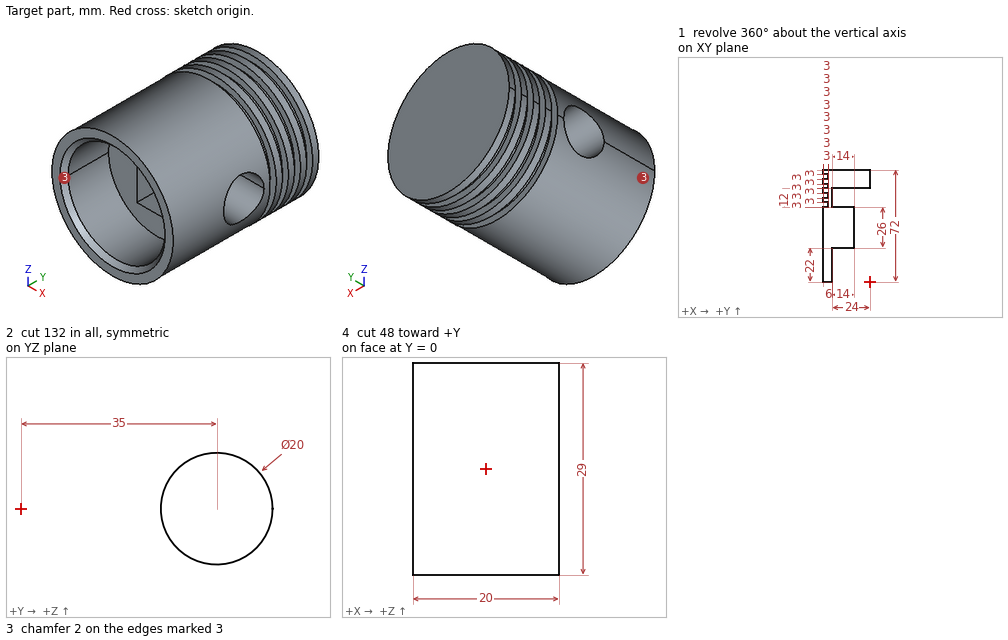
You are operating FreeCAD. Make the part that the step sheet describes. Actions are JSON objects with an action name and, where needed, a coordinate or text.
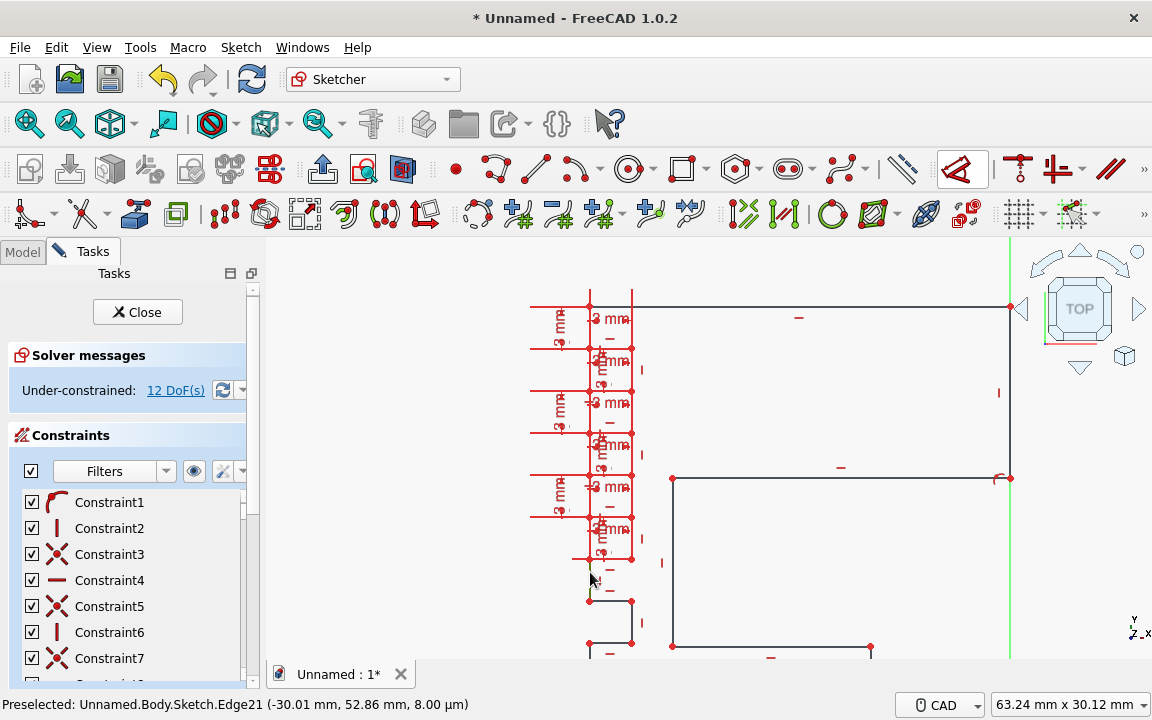
{"action": "key", "text": "i"}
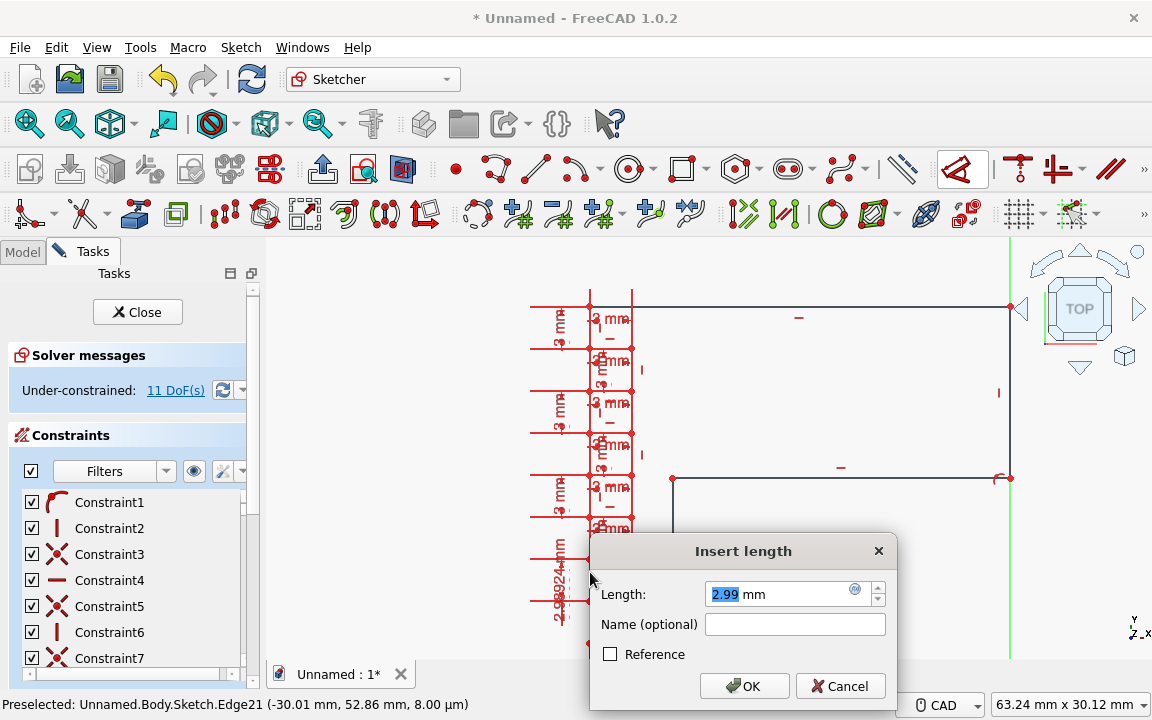
{"action": "type", "text": "3"}
{"action": "key", "text": "Return"}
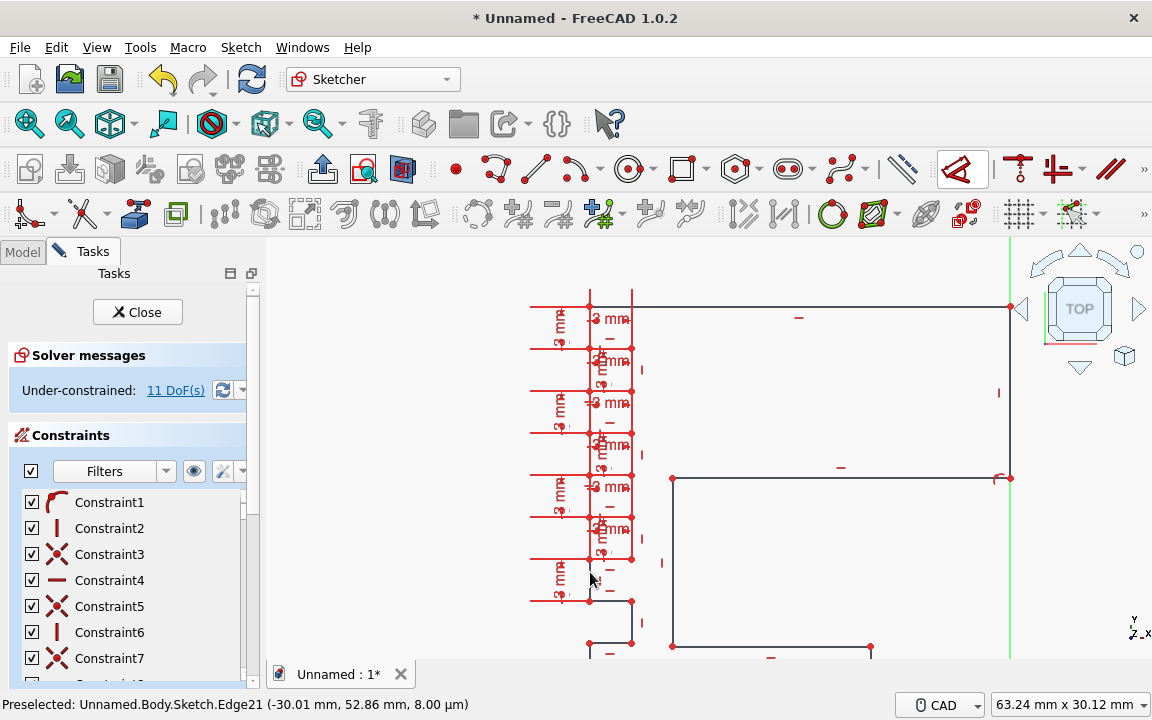
{"action": "left_click", "coordinate": [602, 601]}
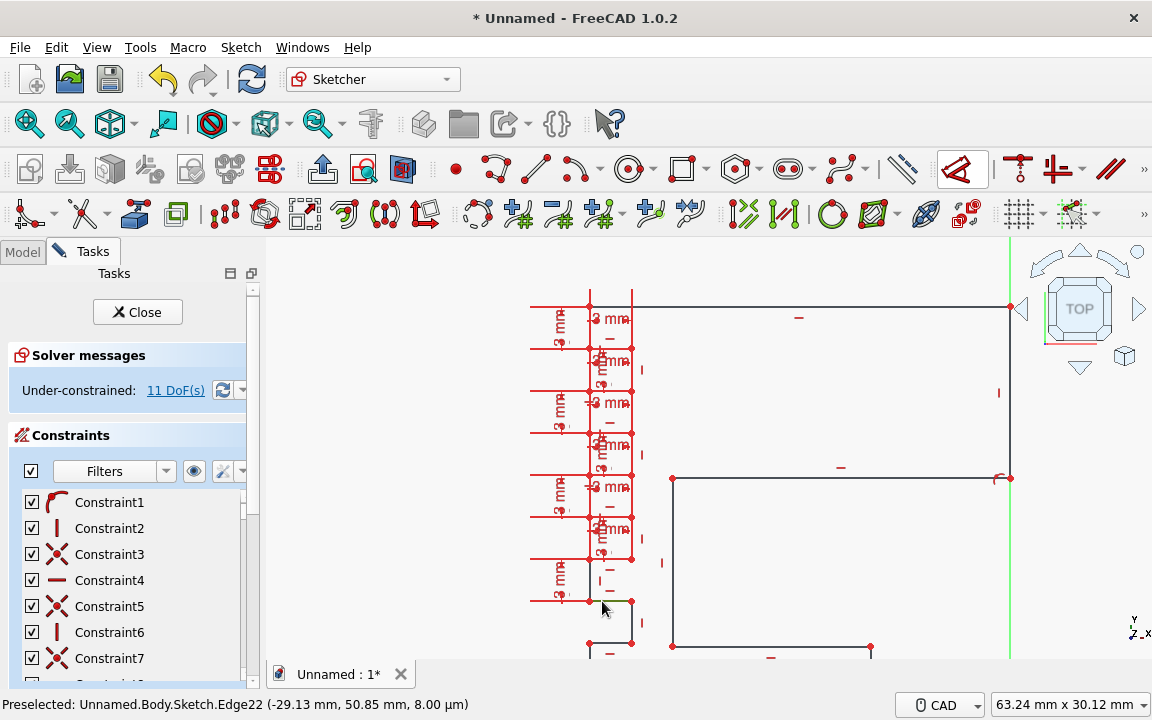
{"action": "key", "text": "l"}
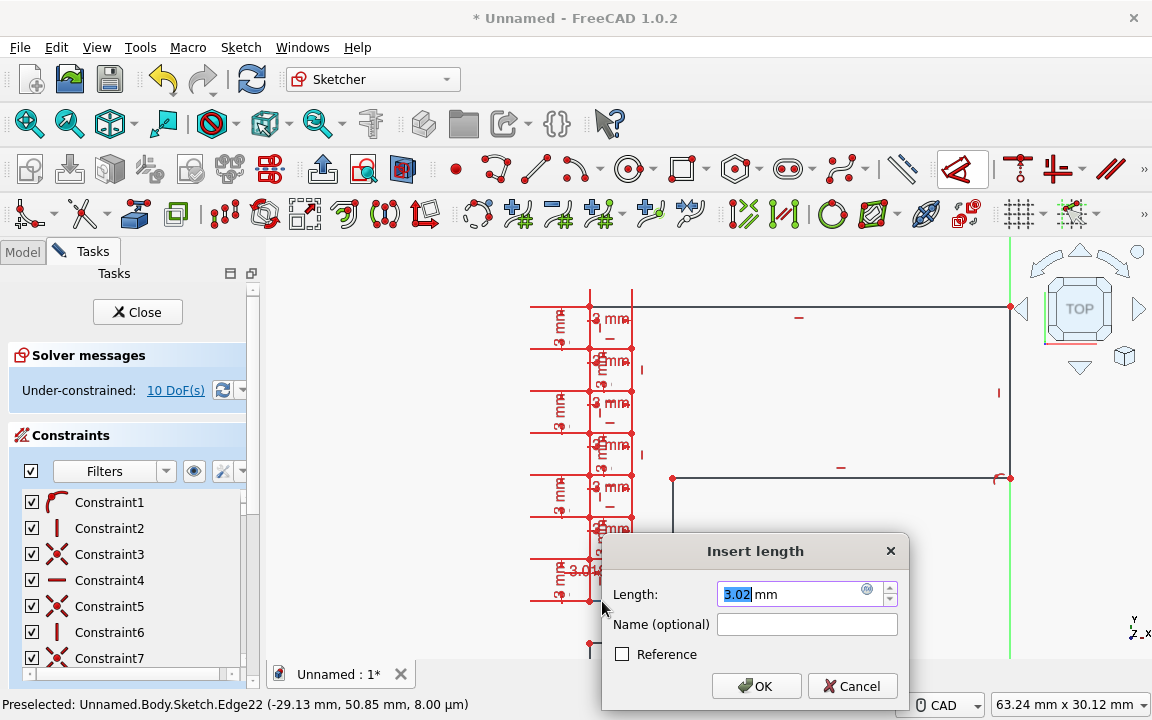
{"action": "type", "text": "3"}
{"action": "key", "text": "Return"}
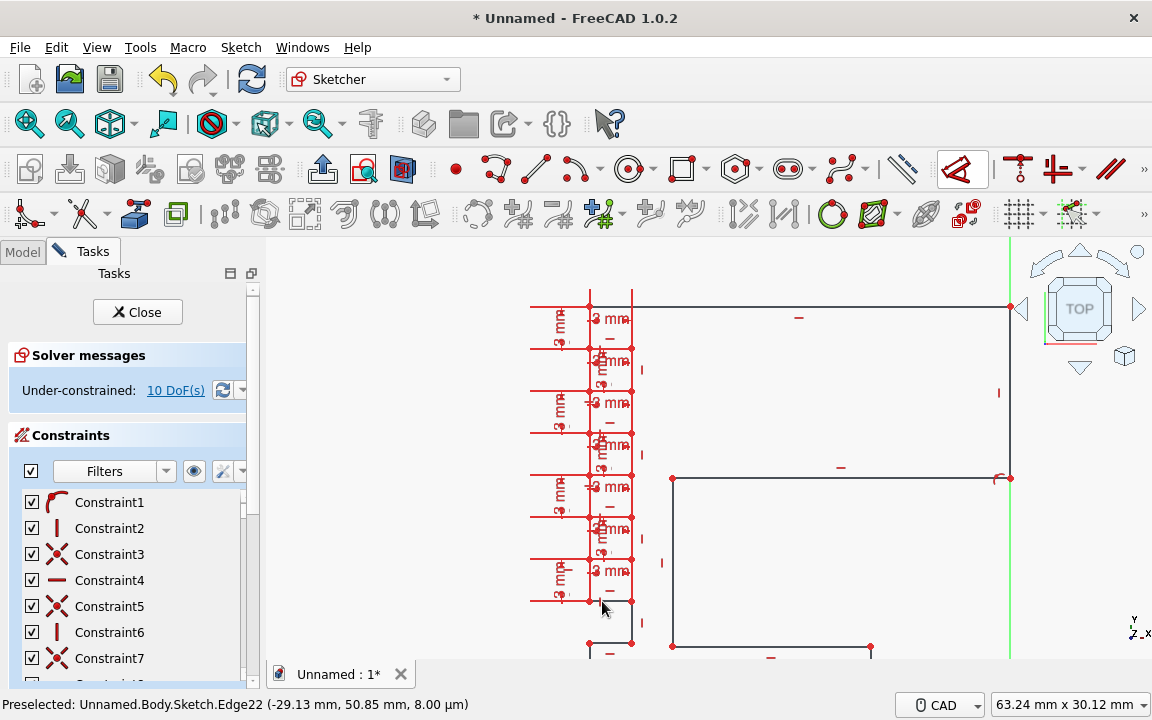
{"action": "left_click", "coordinate": [632, 614]}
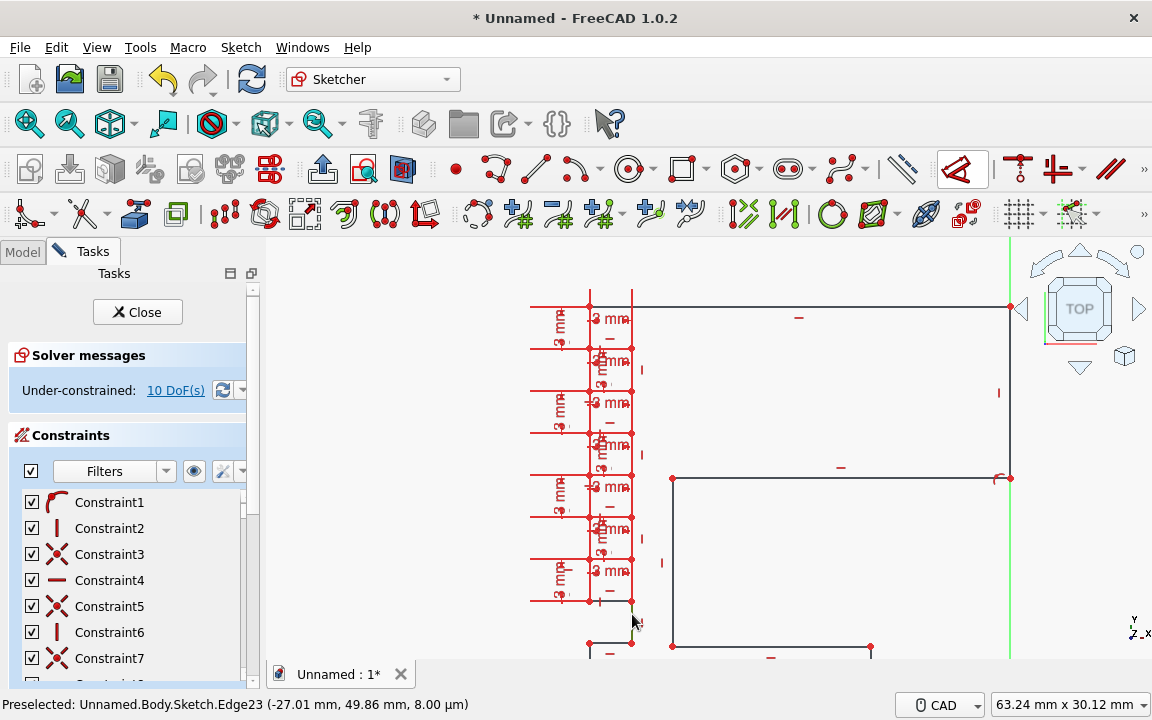
{"action": "left_click", "coordinate": [982, 170]}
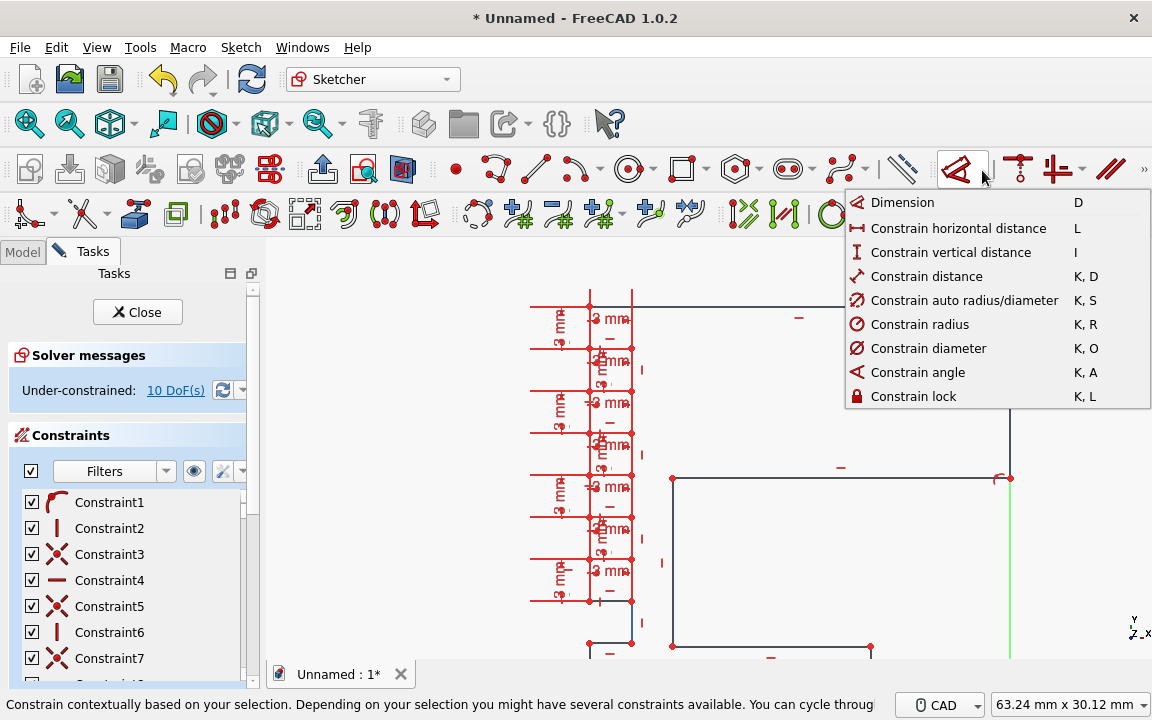
{"action": "left_click", "coordinate": [998, 252]}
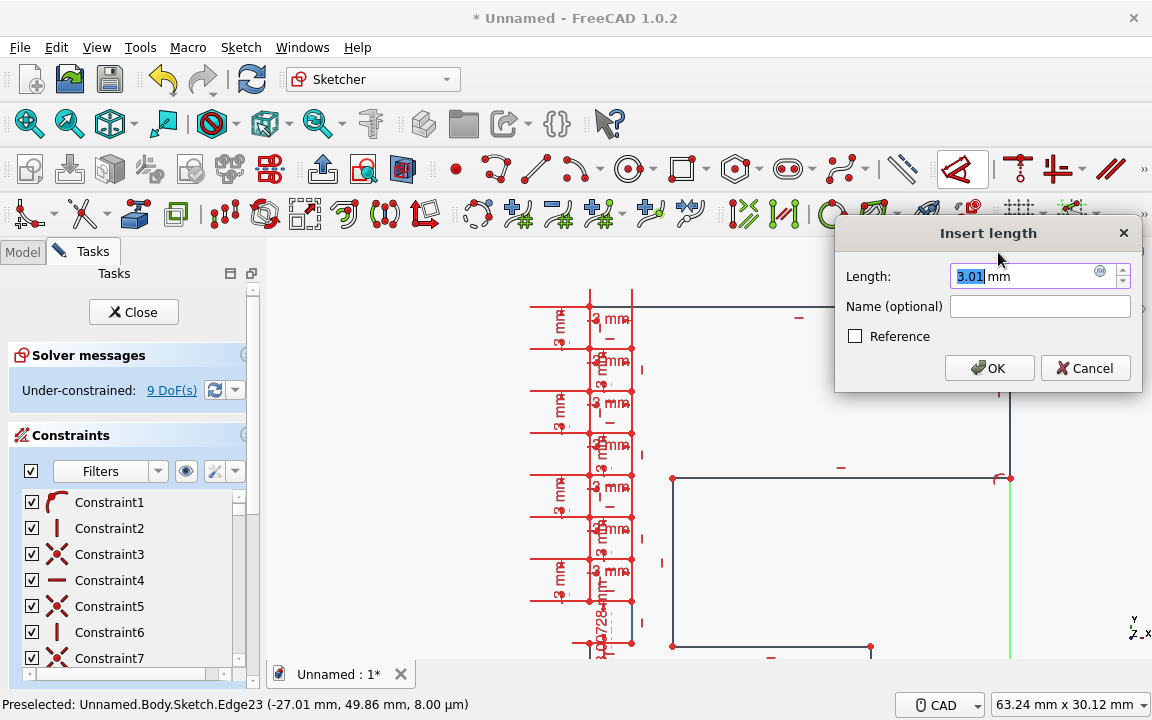
{"action": "type", "text": "3"}
{"action": "key", "text": "Return"}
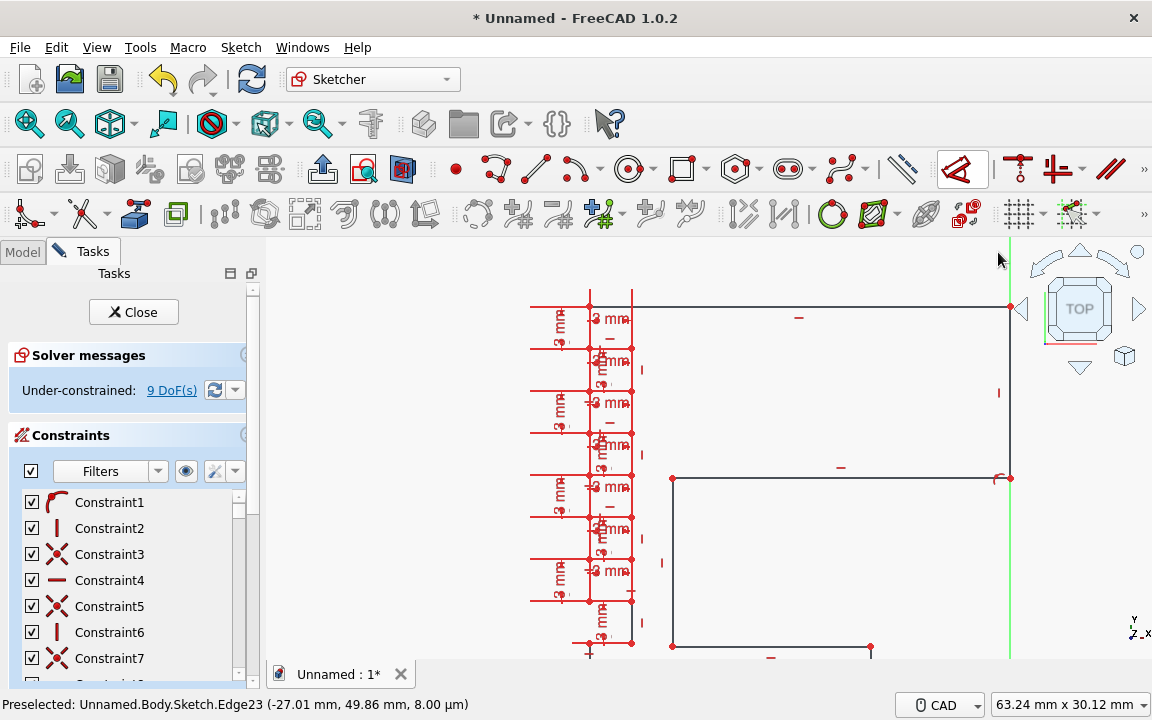
{"action": "scroll", "coordinate": [588, 330], "scroll_direction": "down", "scroll_amount": 7}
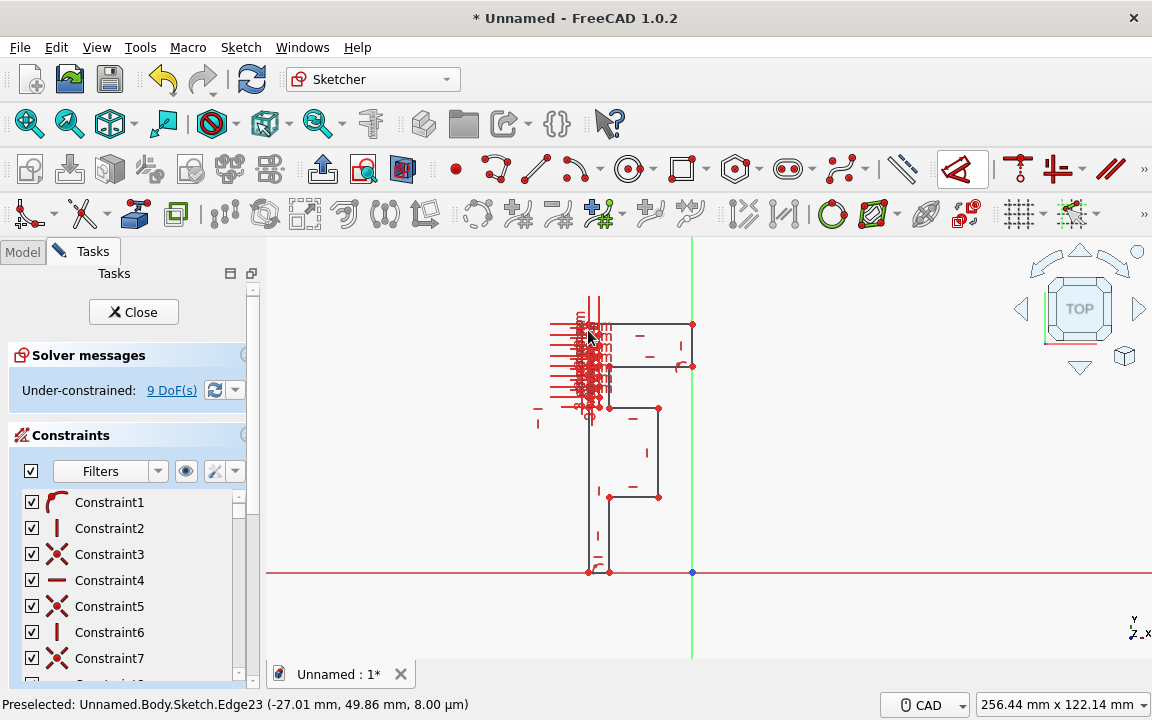
{"action": "scroll", "coordinate": [596, 407], "scroll_direction": "up", "scroll_amount": 8}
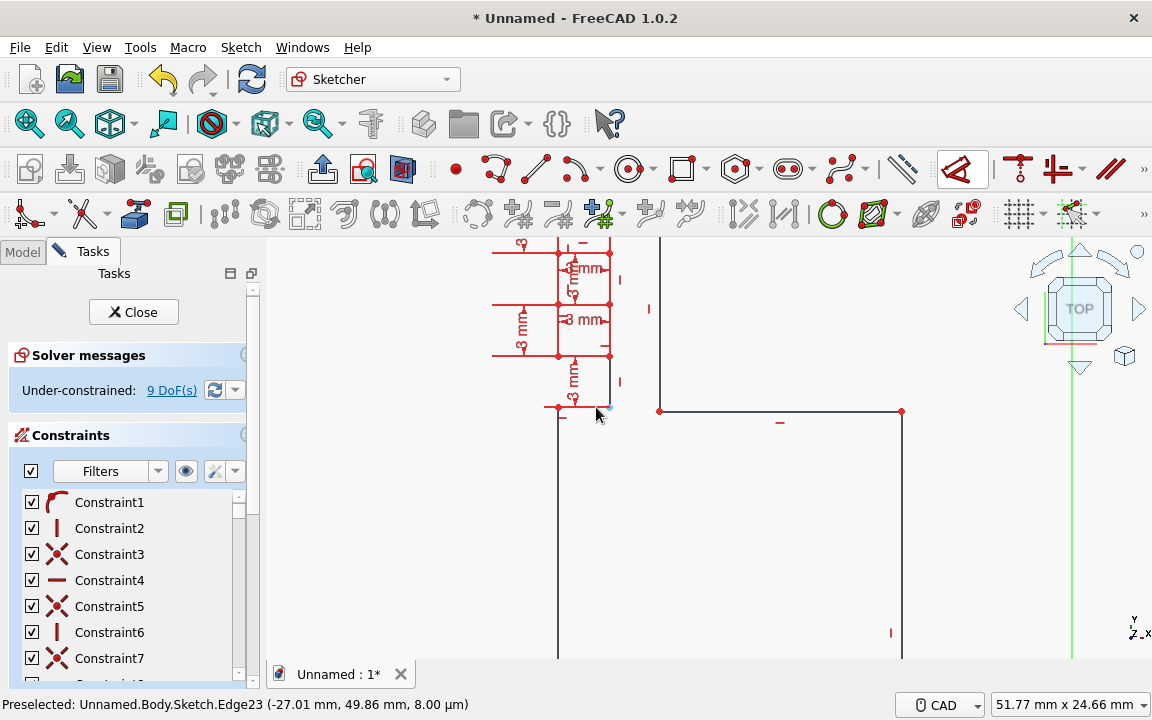
{"action": "left_click", "coordinate": [594, 407]}